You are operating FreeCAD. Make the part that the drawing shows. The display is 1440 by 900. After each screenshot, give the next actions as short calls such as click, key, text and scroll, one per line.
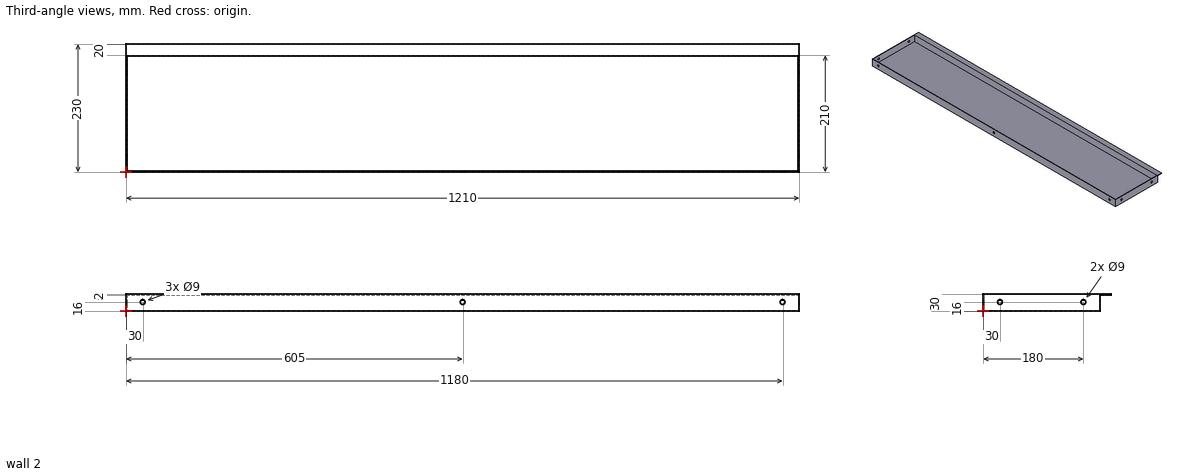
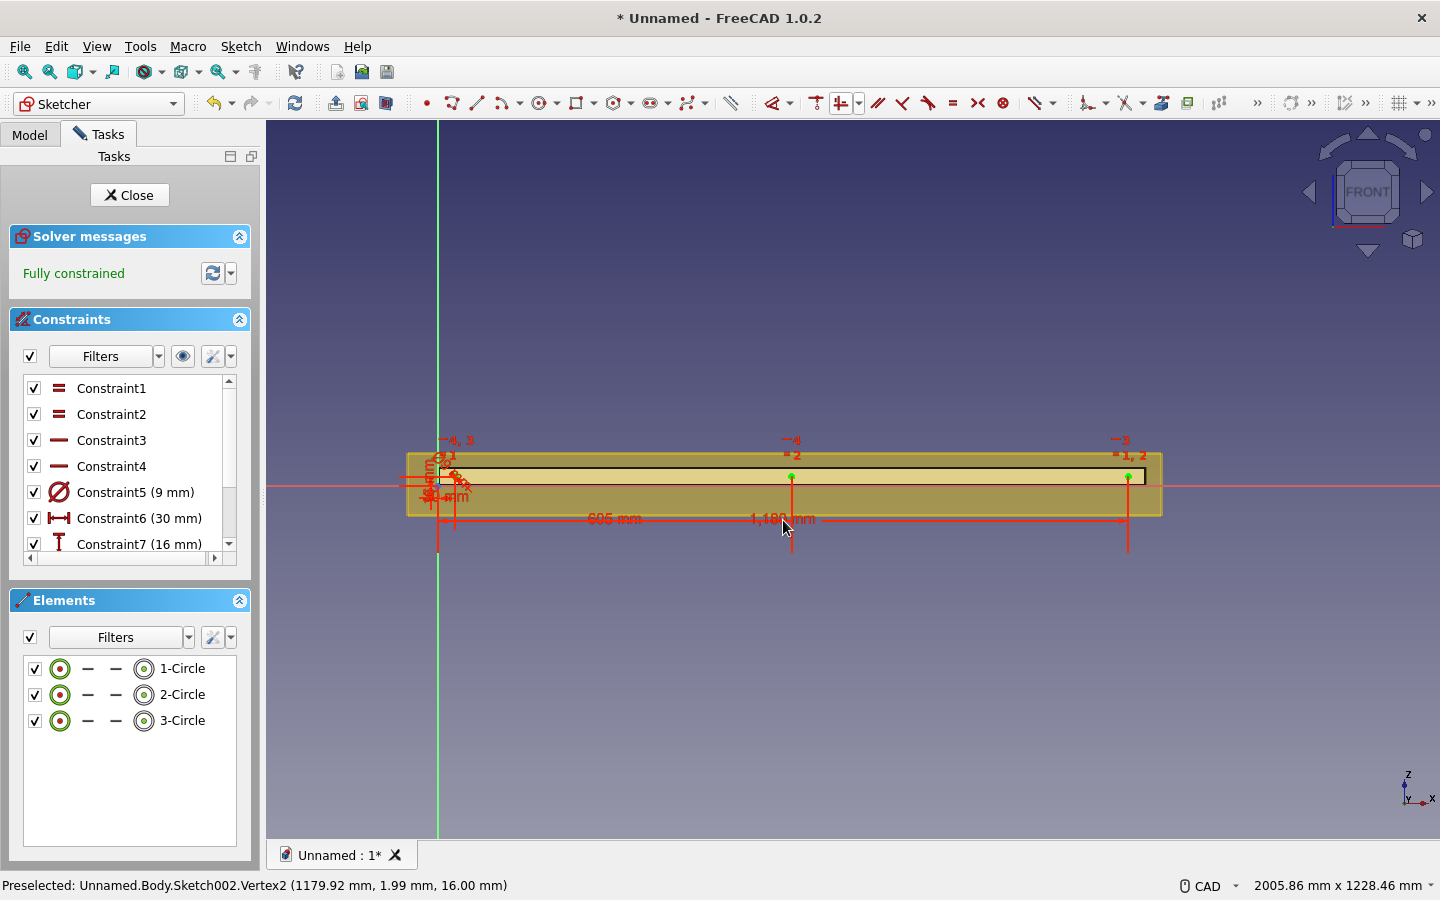
click(130, 195)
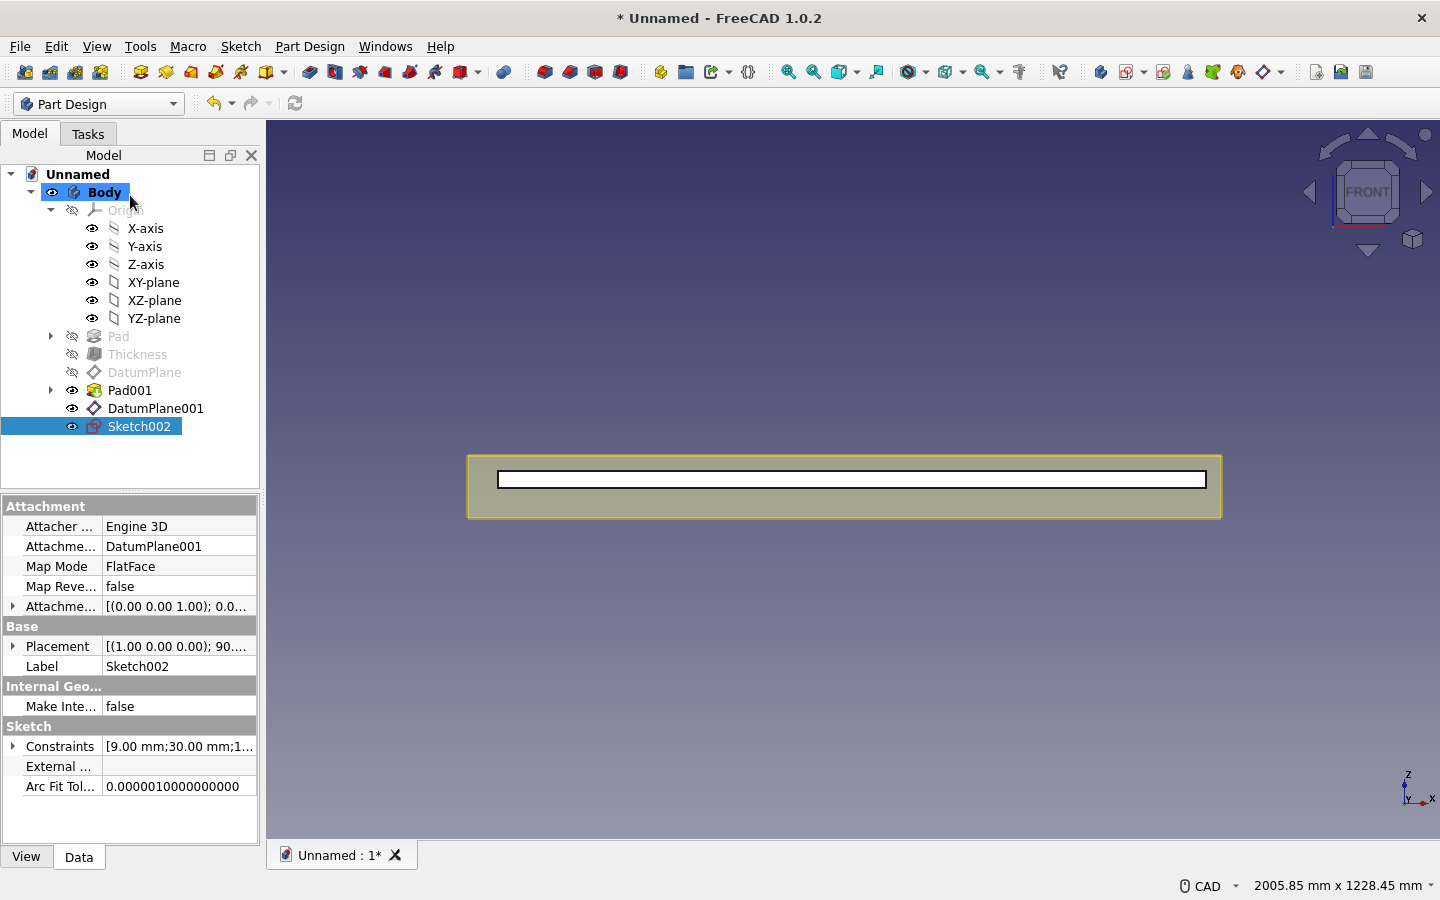
click(310, 72)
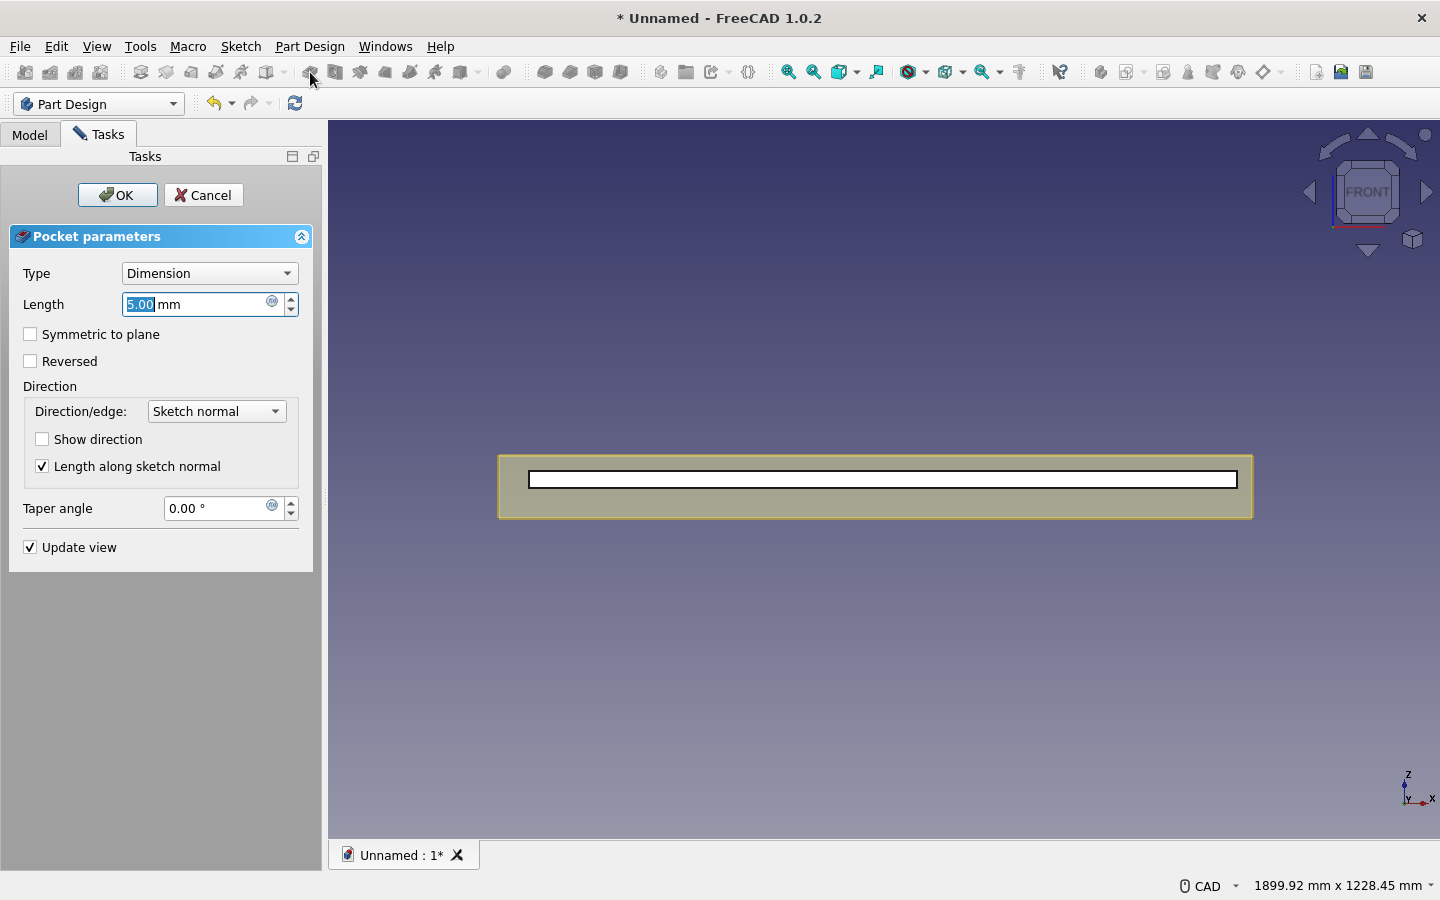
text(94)
key(Tab)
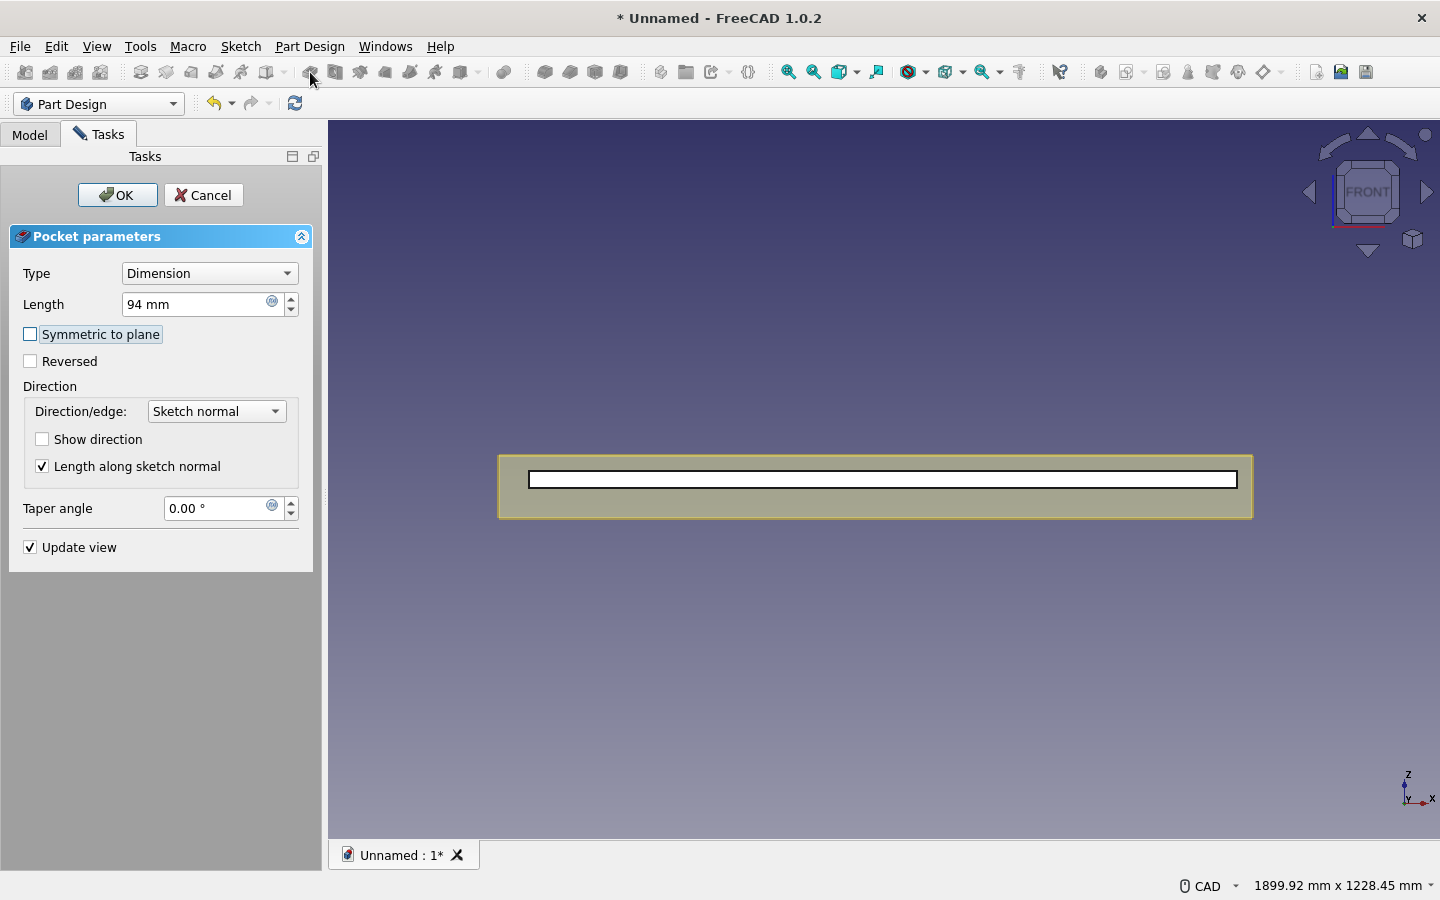
click(31, 361)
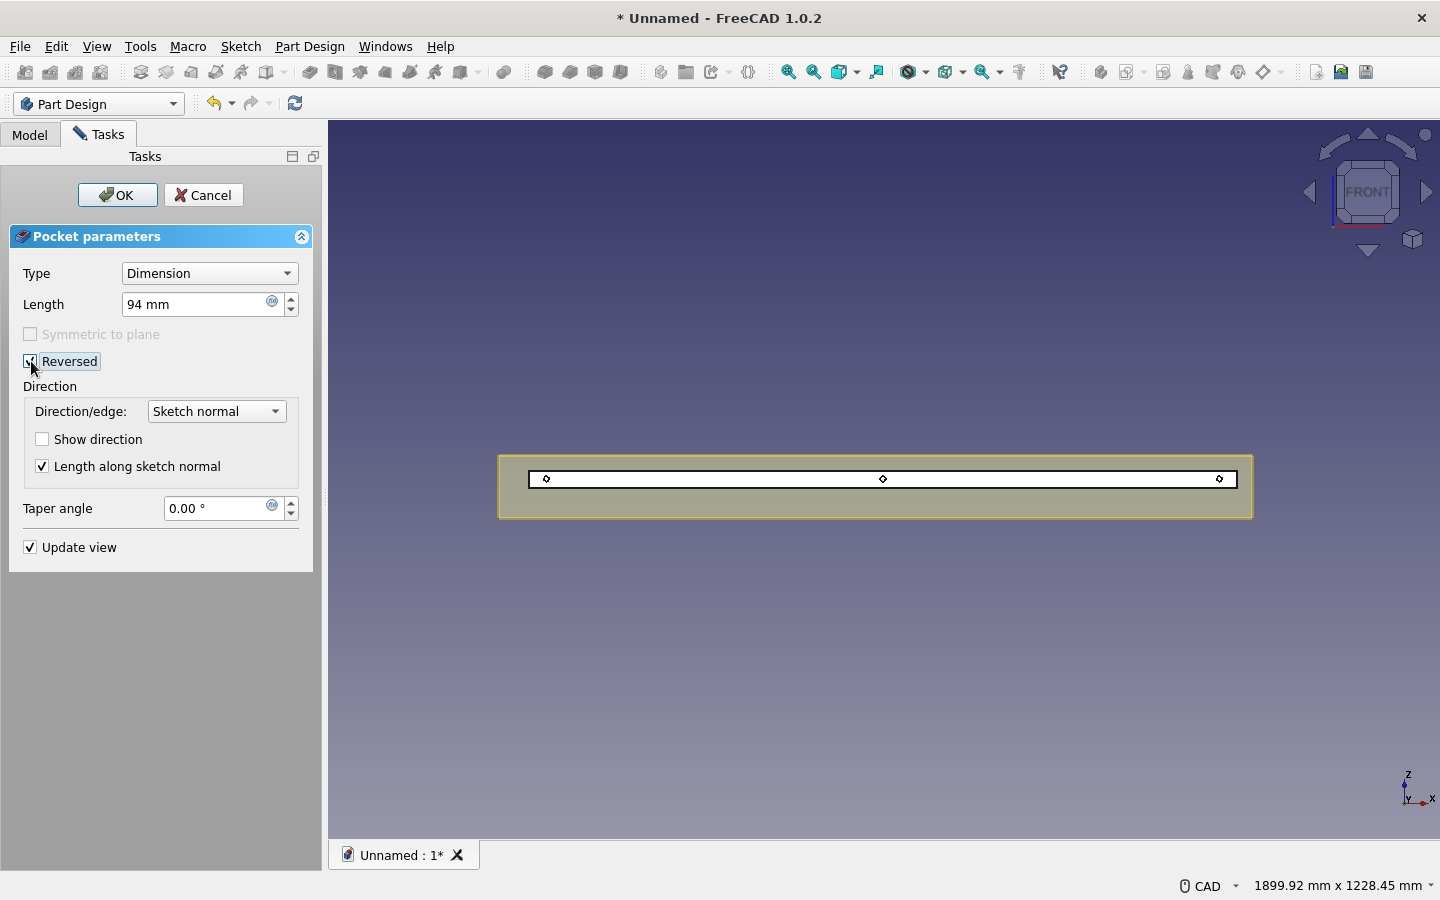
click(118, 195)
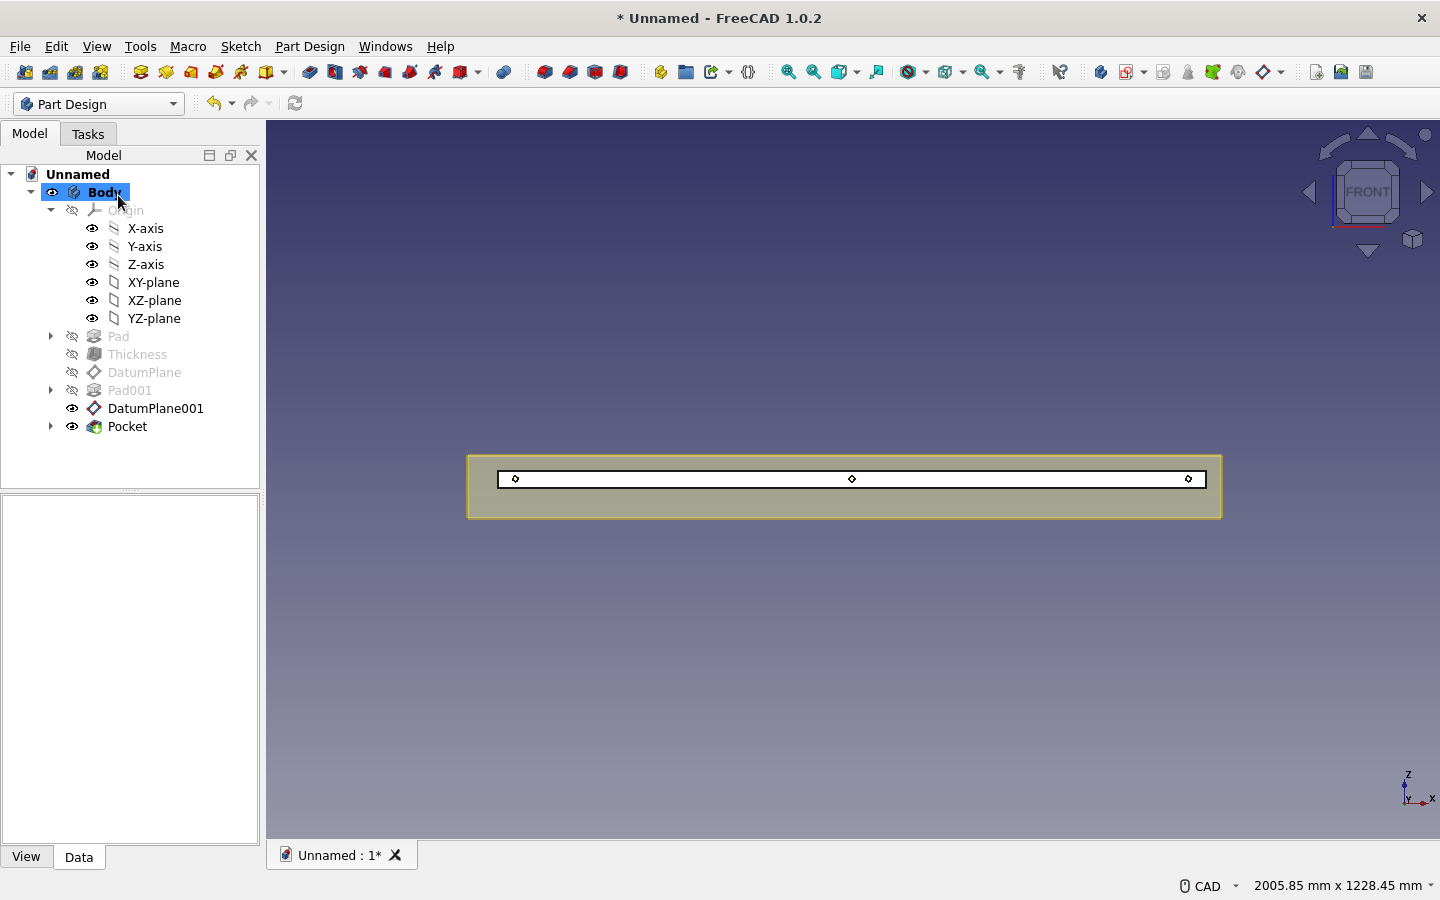
click(117, 408)
key(space)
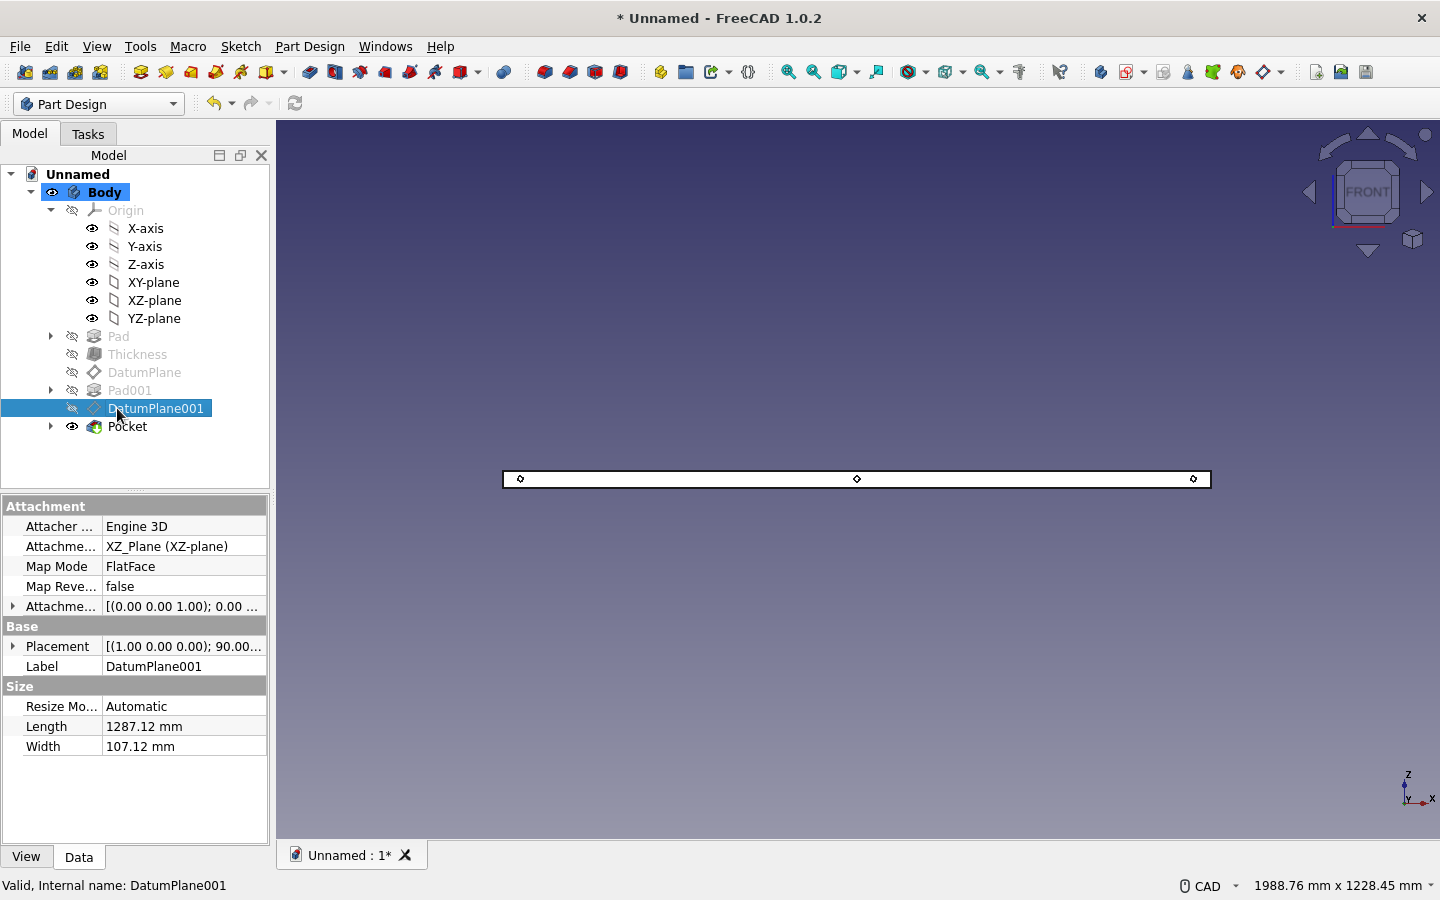
click(137, 318)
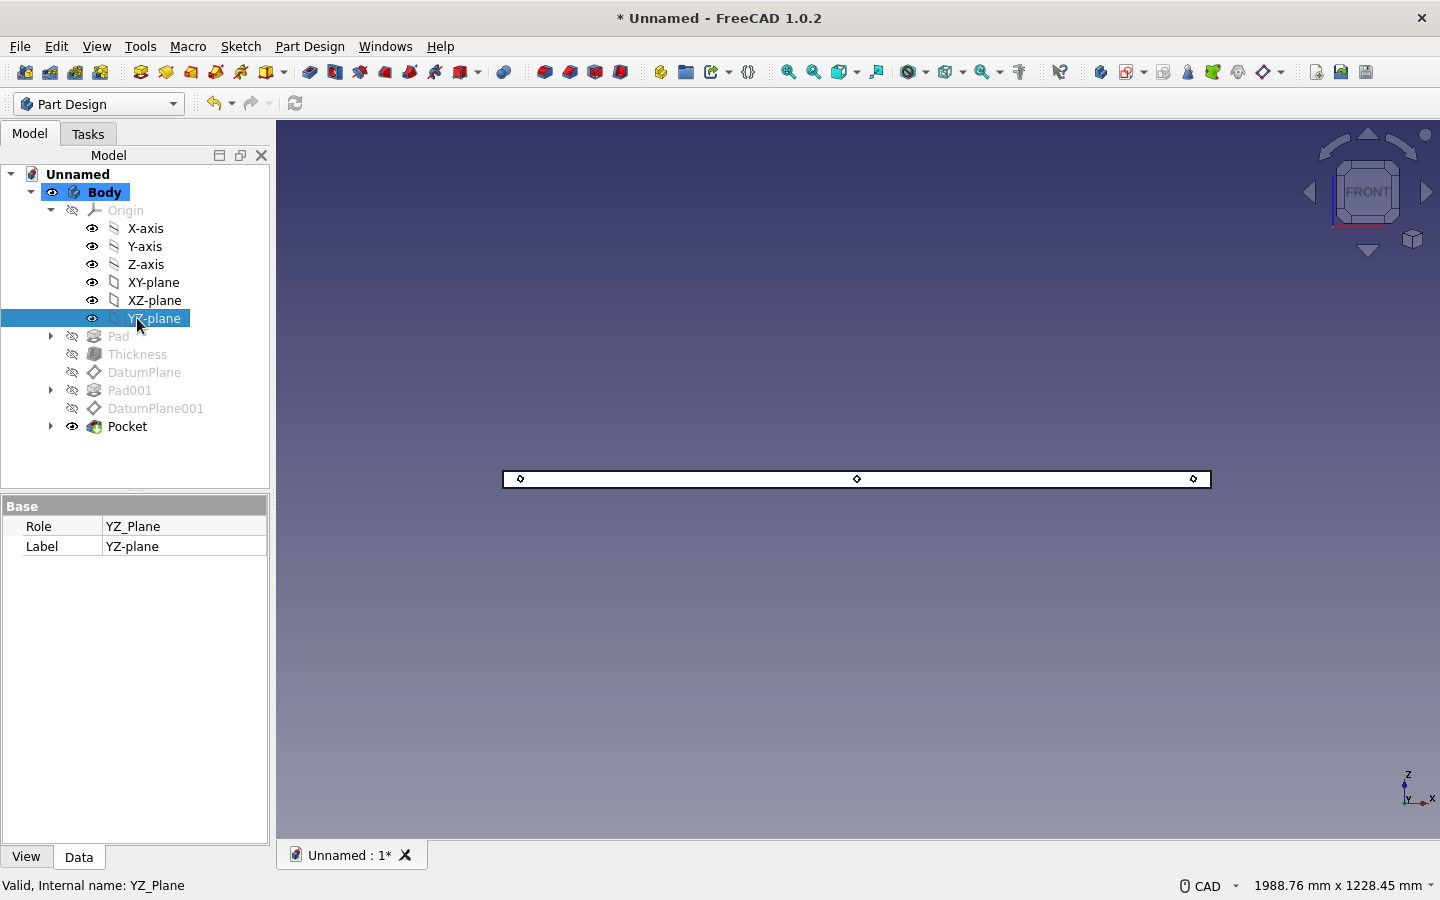
click(1262, 72)